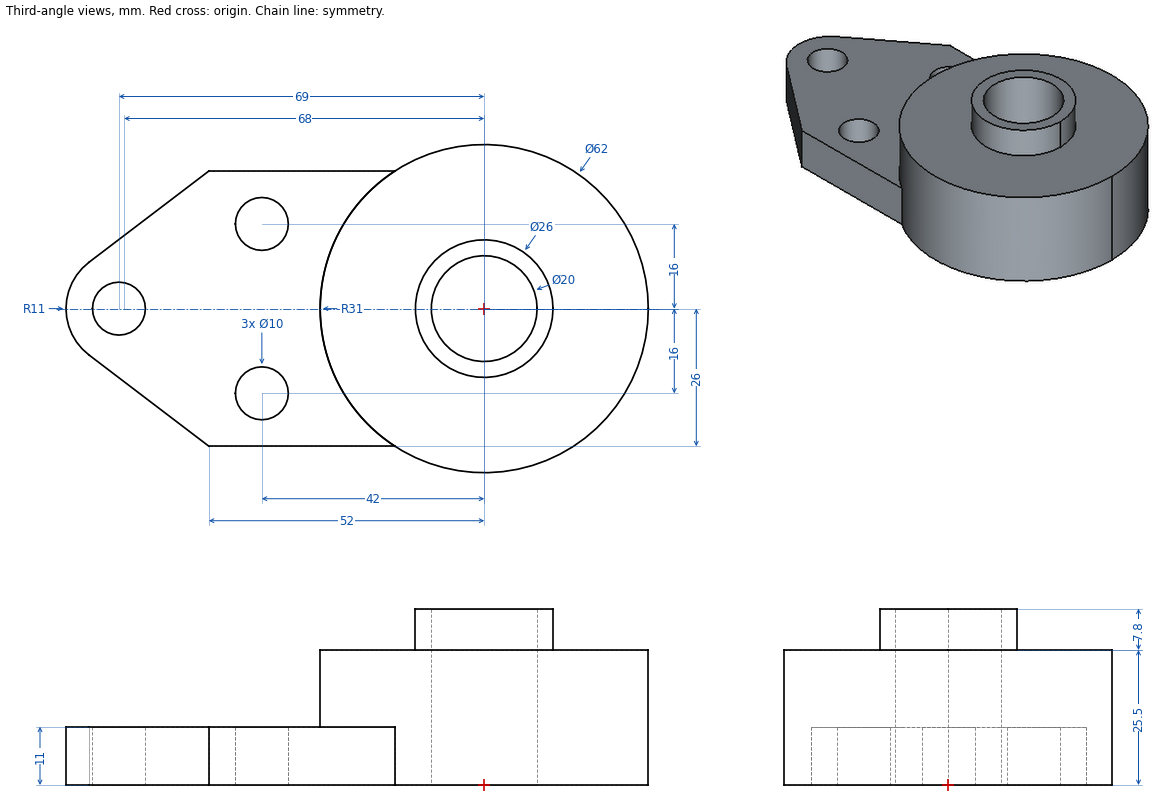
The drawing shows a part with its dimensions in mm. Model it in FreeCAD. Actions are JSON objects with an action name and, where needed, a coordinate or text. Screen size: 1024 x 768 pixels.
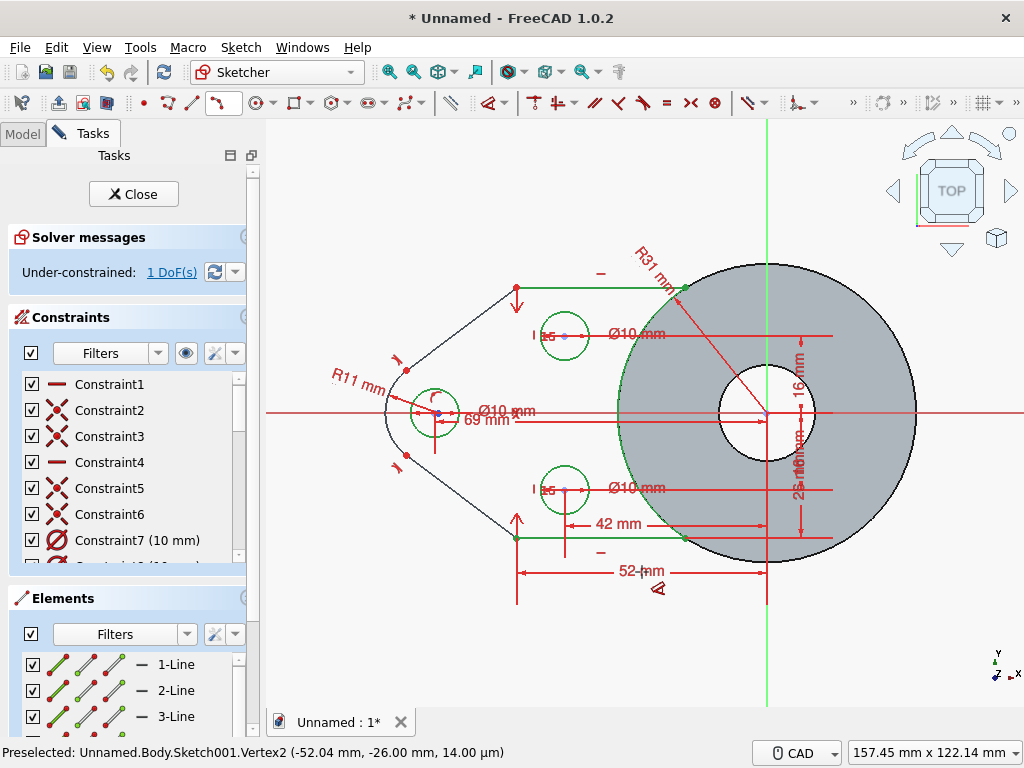
{"action": "scroll", "coordinate": [438, 413], "scroll_direction": "up", "scroll_amount": 7}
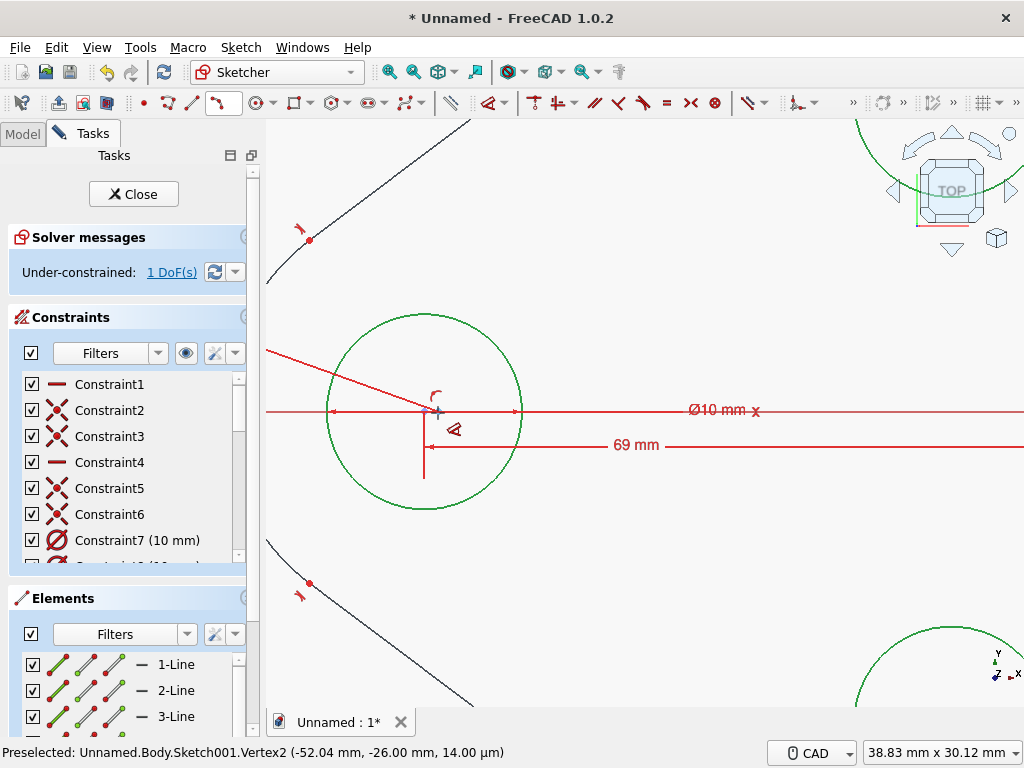
{"action": "left_click", "coordinate": [439, 412]}
{"action": "left_click", "coordinate": [552, 446]}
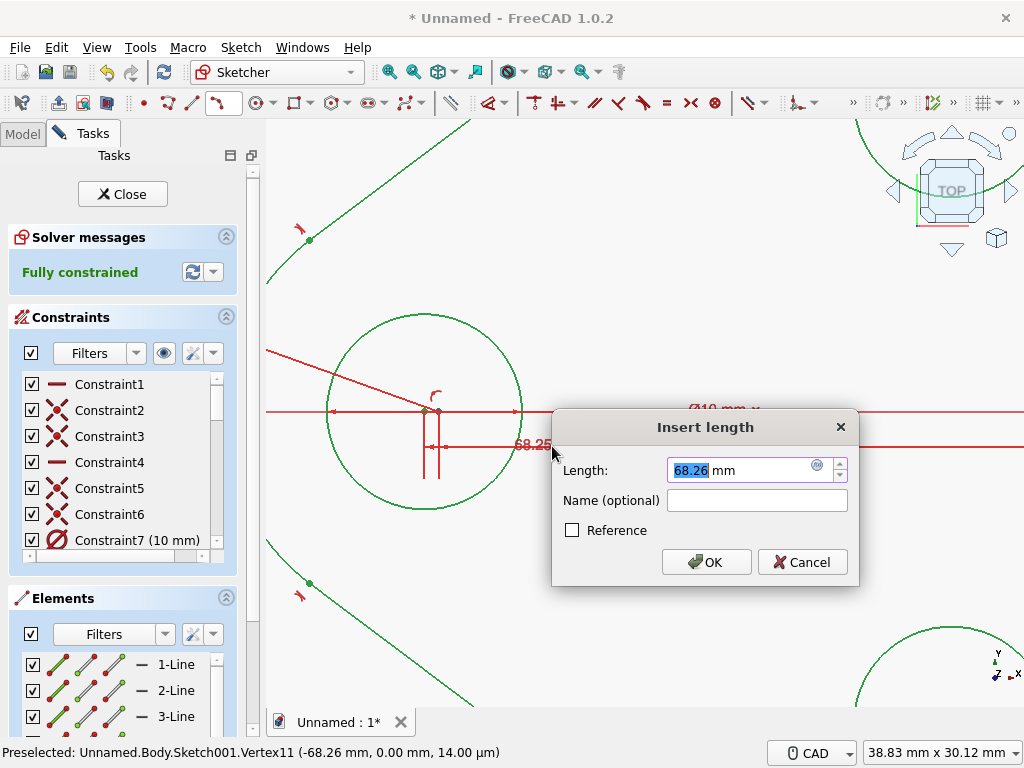
{"action": "type", "text": "68"}
{"action": "key", "text": "Return"}
{"action": "key", "text": "Escape"}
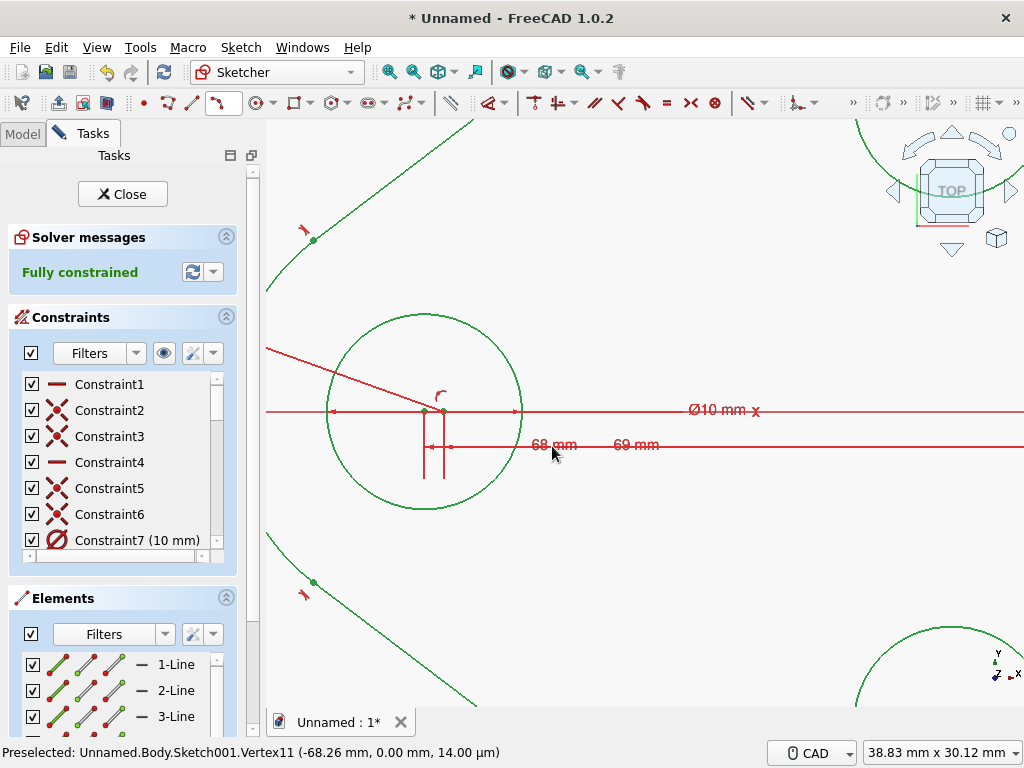
{"action": "left_click", "coordinate": [123, 194]}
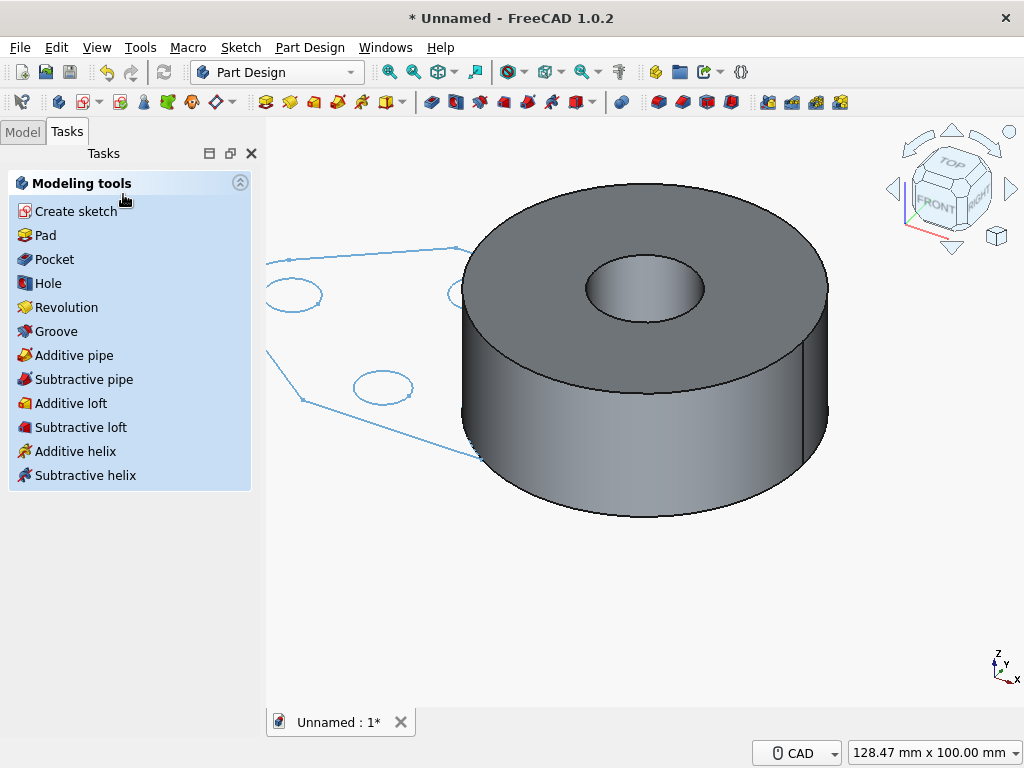
{"action": "left_click", "coordinate": [266, 102]}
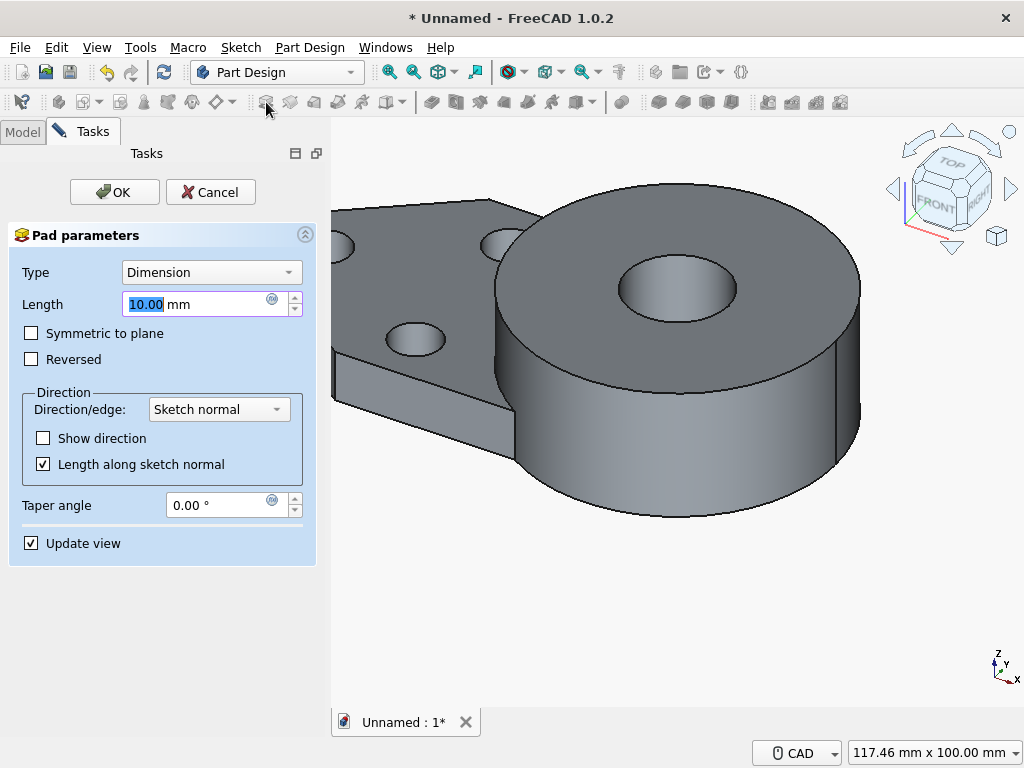
{"action": "type", "text": "11"}
{"action": "key", "text": "Tab"}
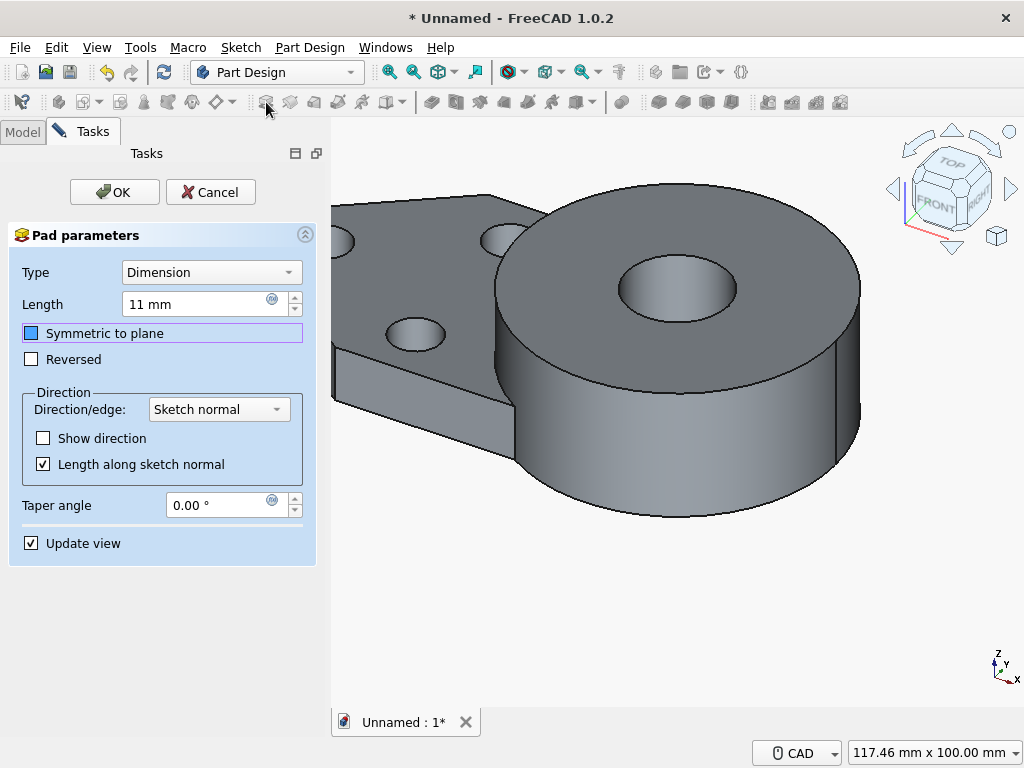
{"action": "left_click", "coordinate": [115, 192]}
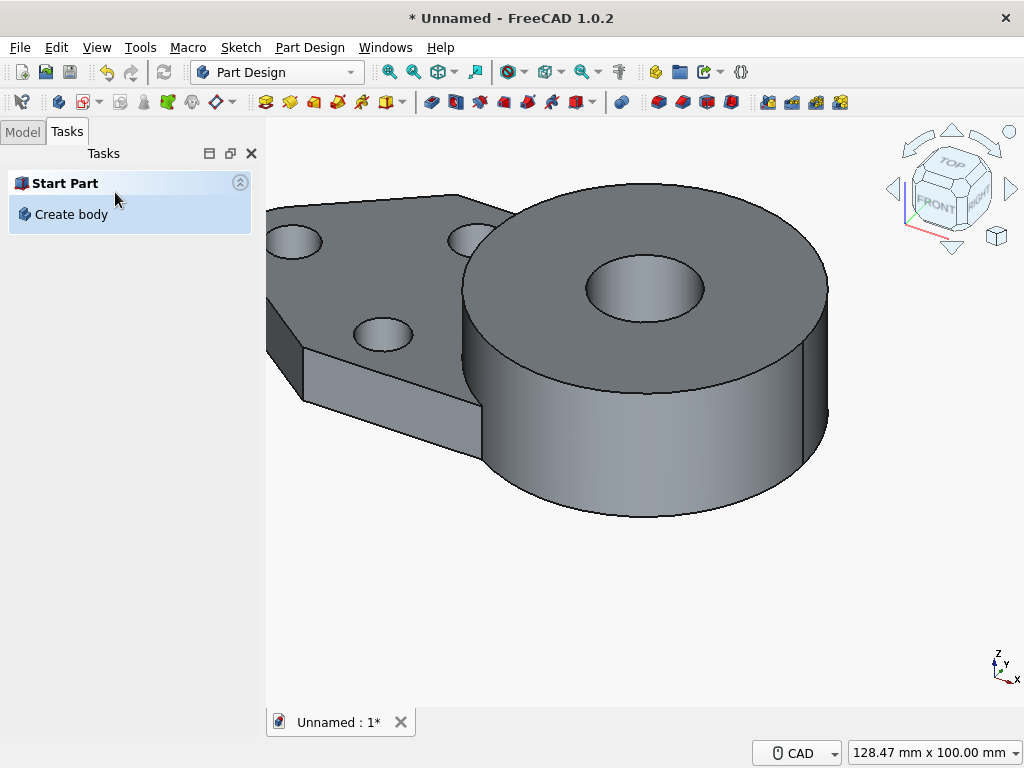
{"action": "left_click", "coordinate": [390, 72]}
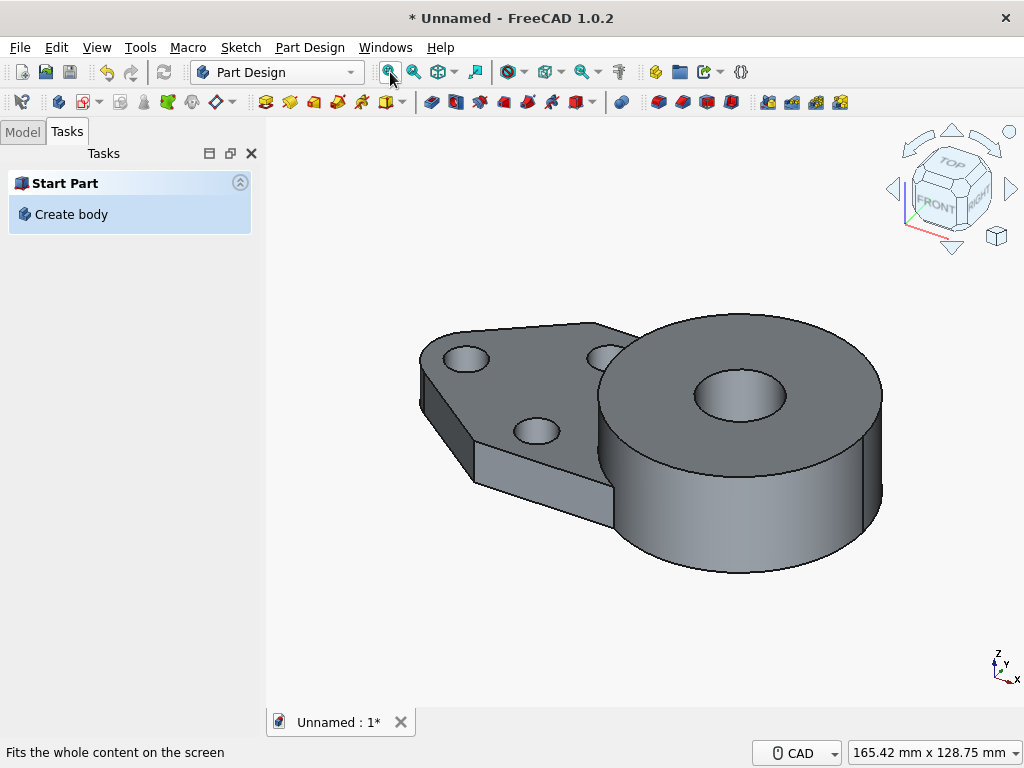
{"action": "left_click", "coordinate": [746, 343]}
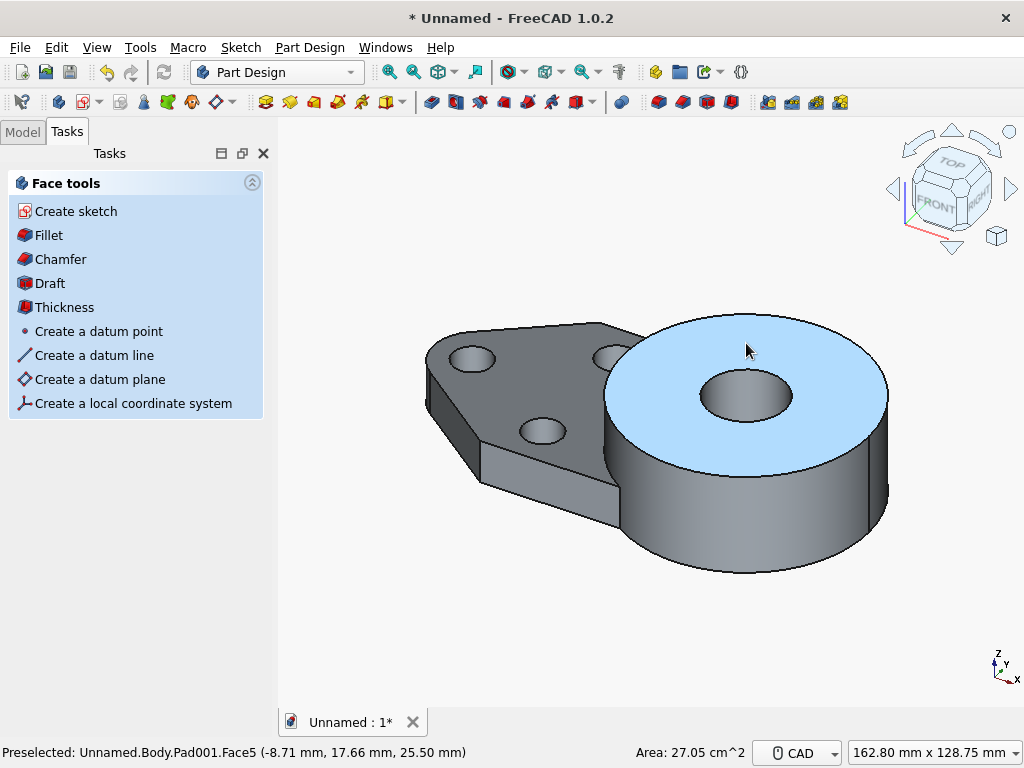
{"action": "left_click", "coordinate": [84, 102]}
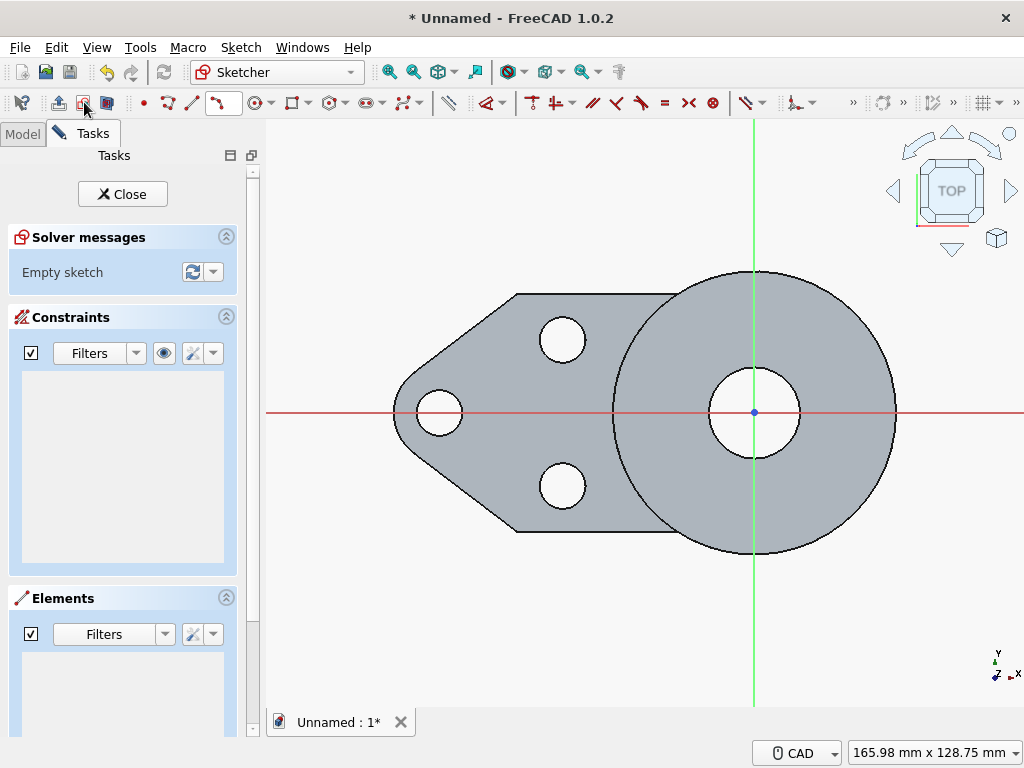
{"action": "scroll", "coordinate": [831, 413], "scroll_direction": "up", "scroll_amount": 6}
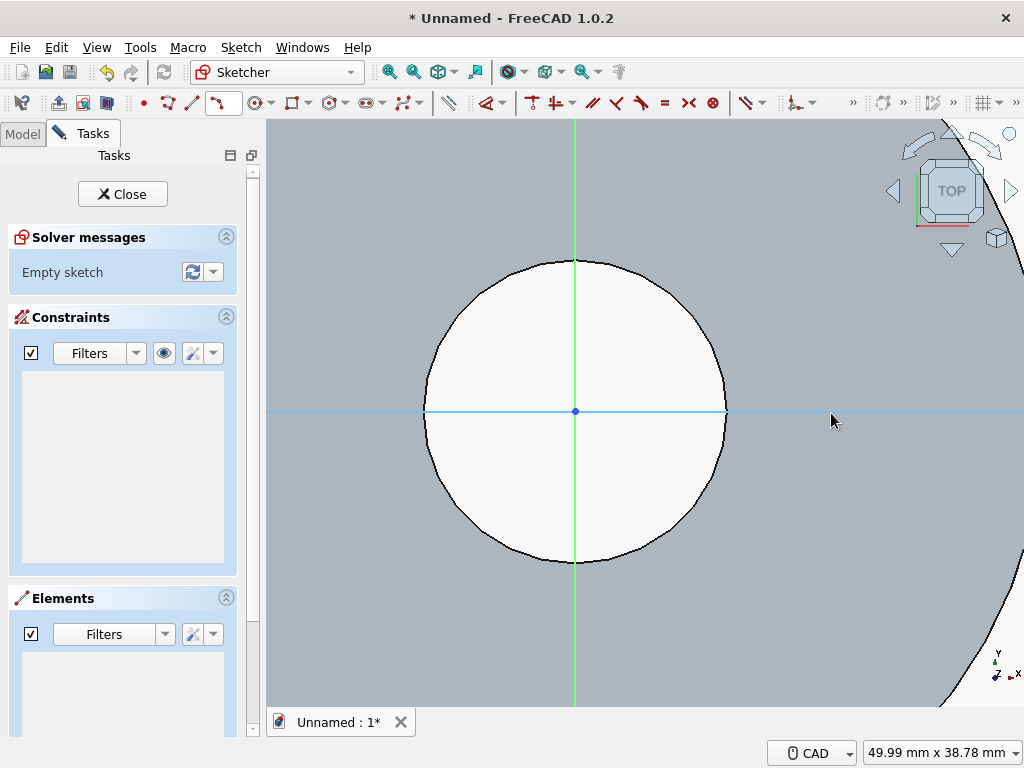
{"action": "left_click", "coordinate": [256, 104]}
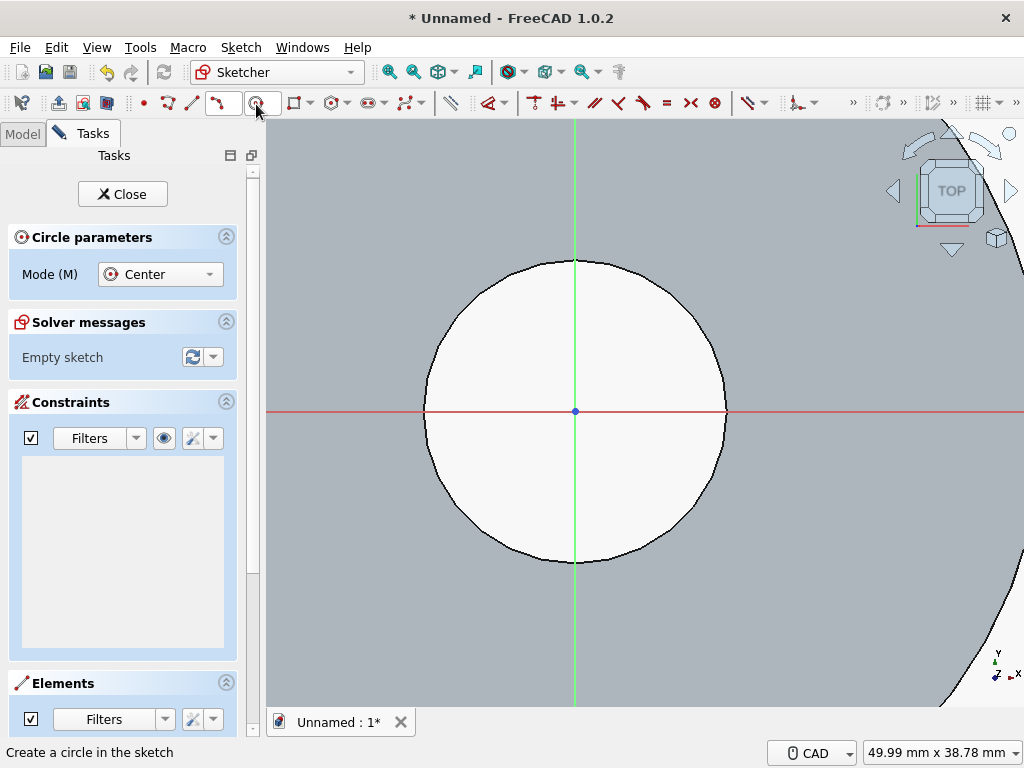
{"action": "left_click", "coordinate": [575, 412]}
{"action": "mouse_move", "coordinate": [715, 272]}